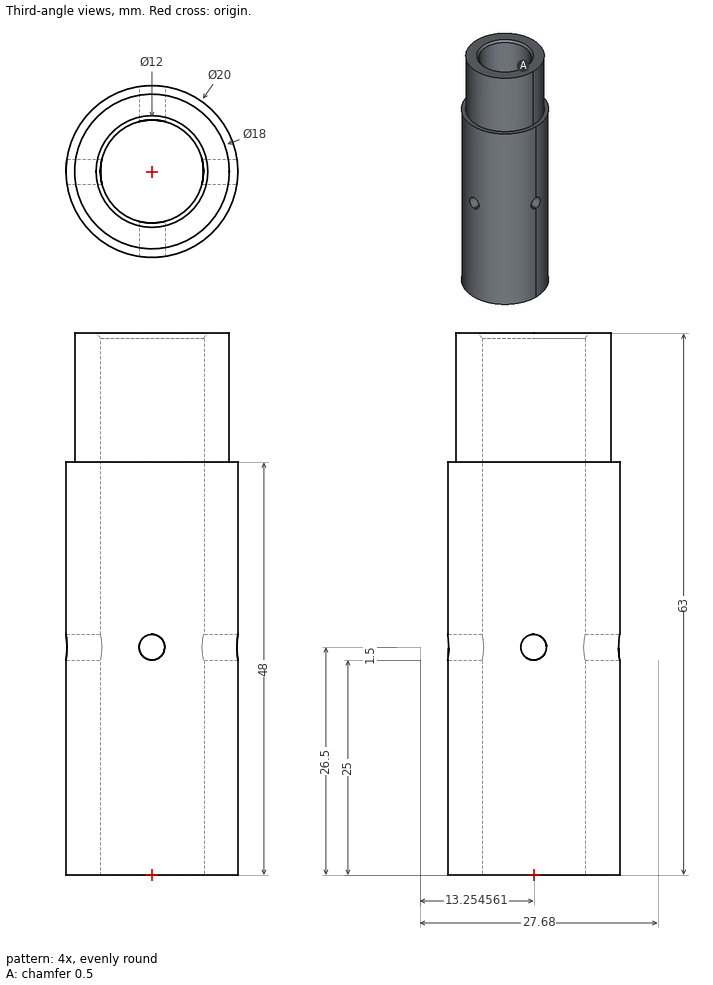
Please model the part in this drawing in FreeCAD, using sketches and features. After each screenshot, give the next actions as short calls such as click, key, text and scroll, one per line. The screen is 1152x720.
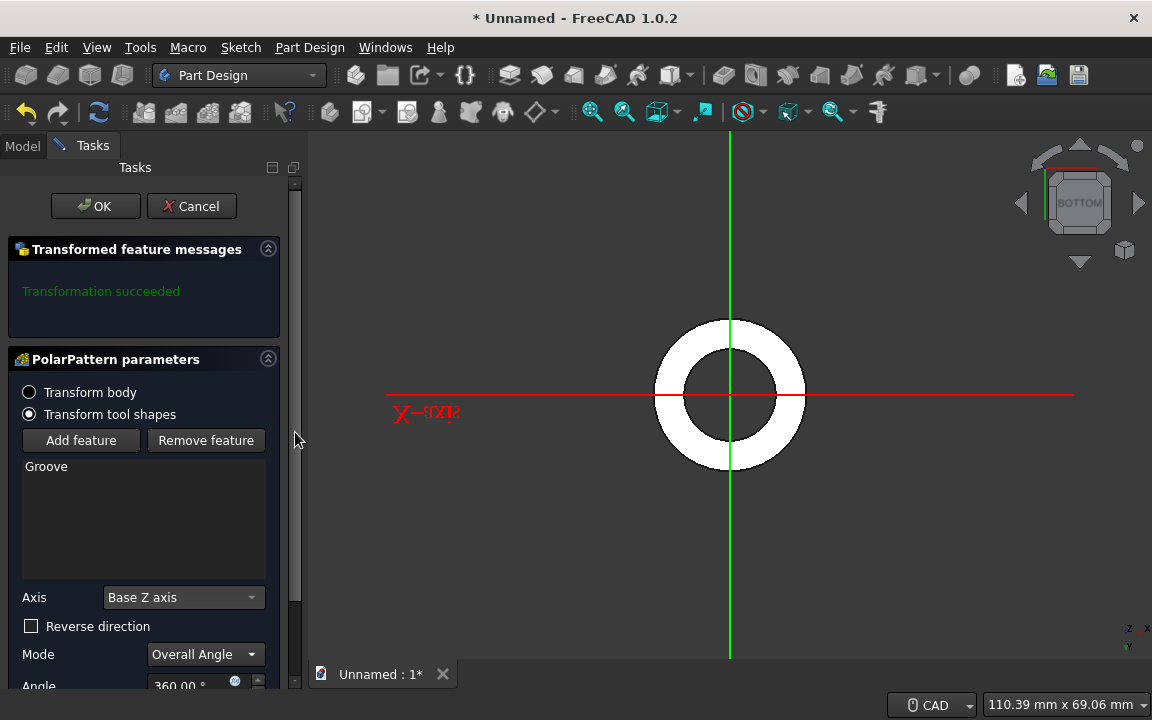
click(96, 206)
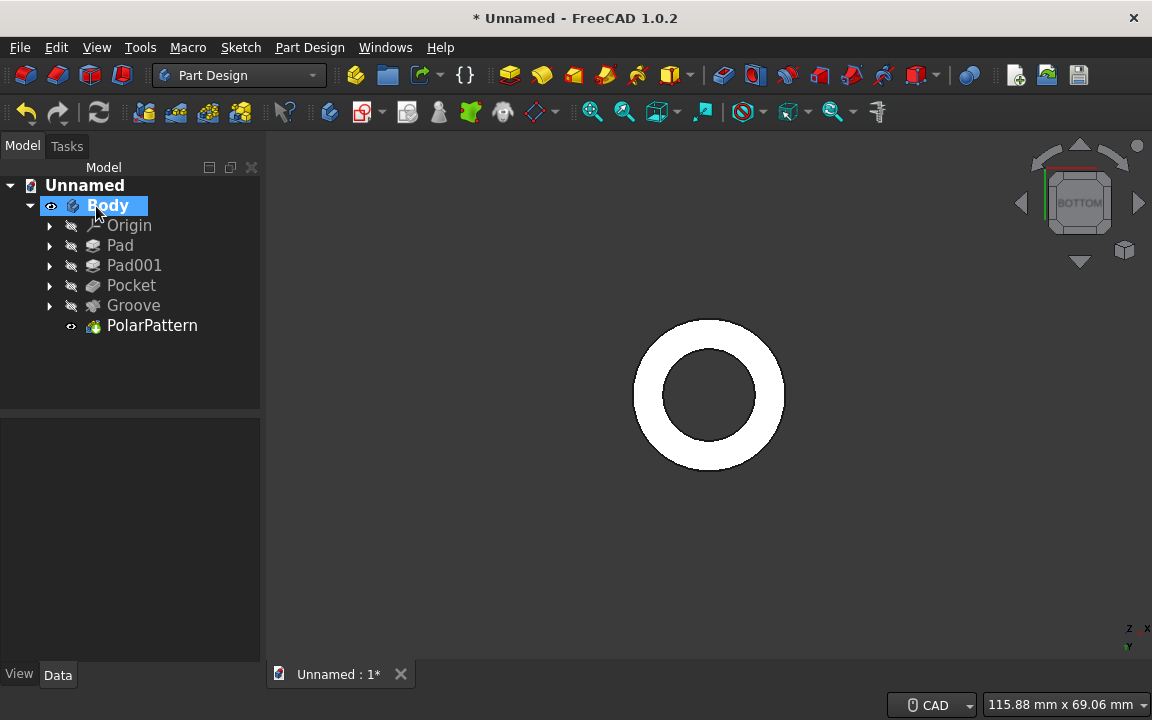
click(594, 112)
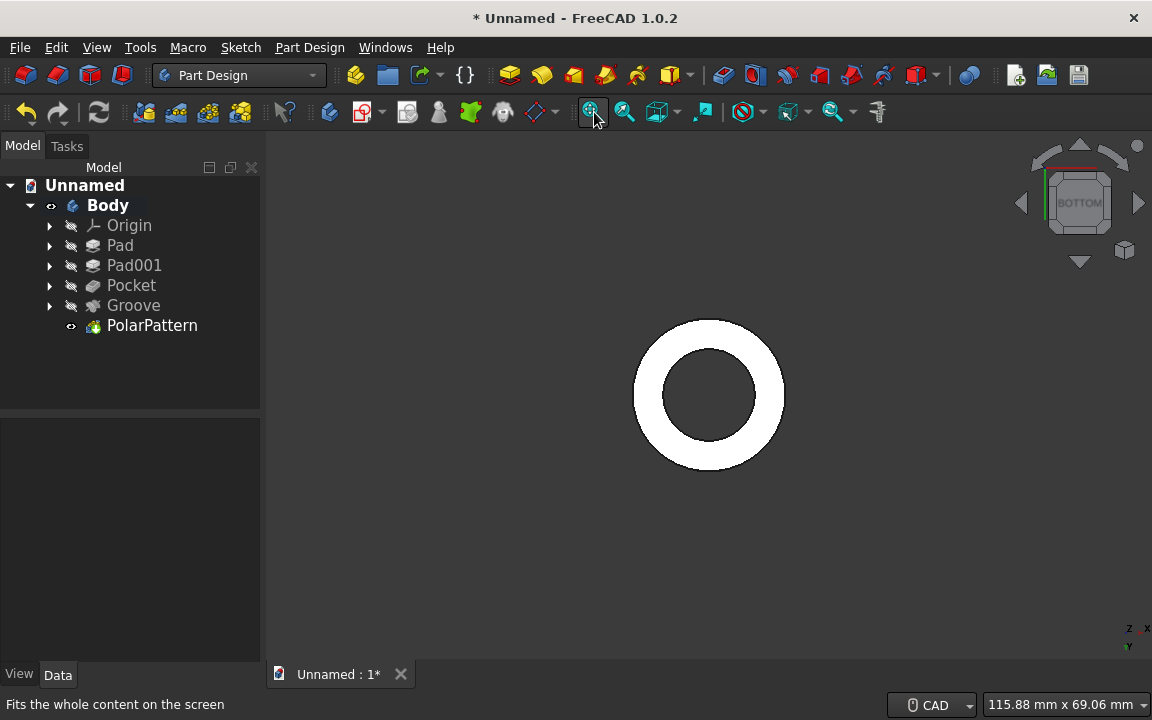
key(0)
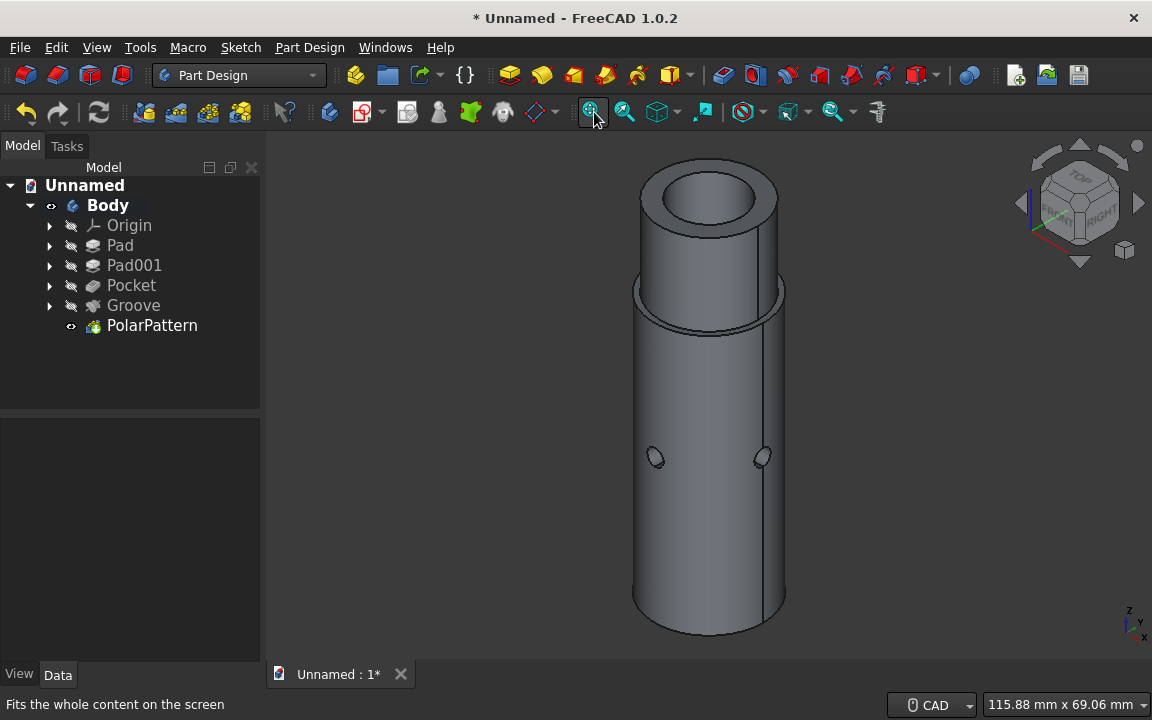
click(677, 179)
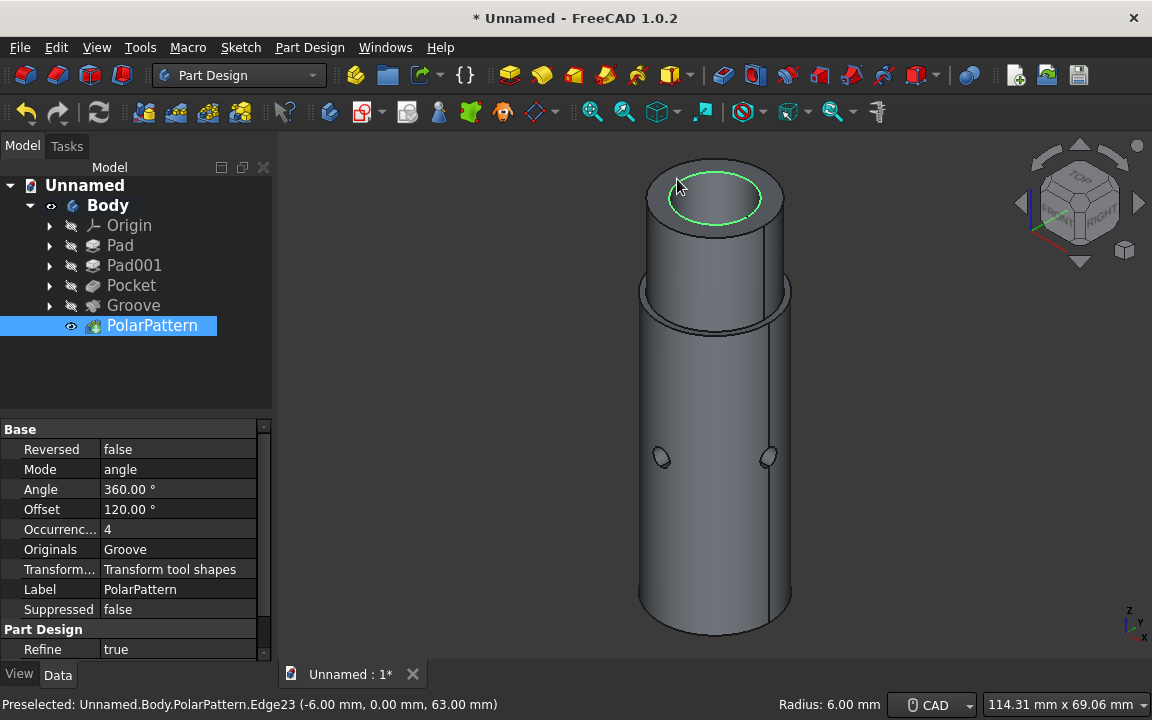
click(58, 76)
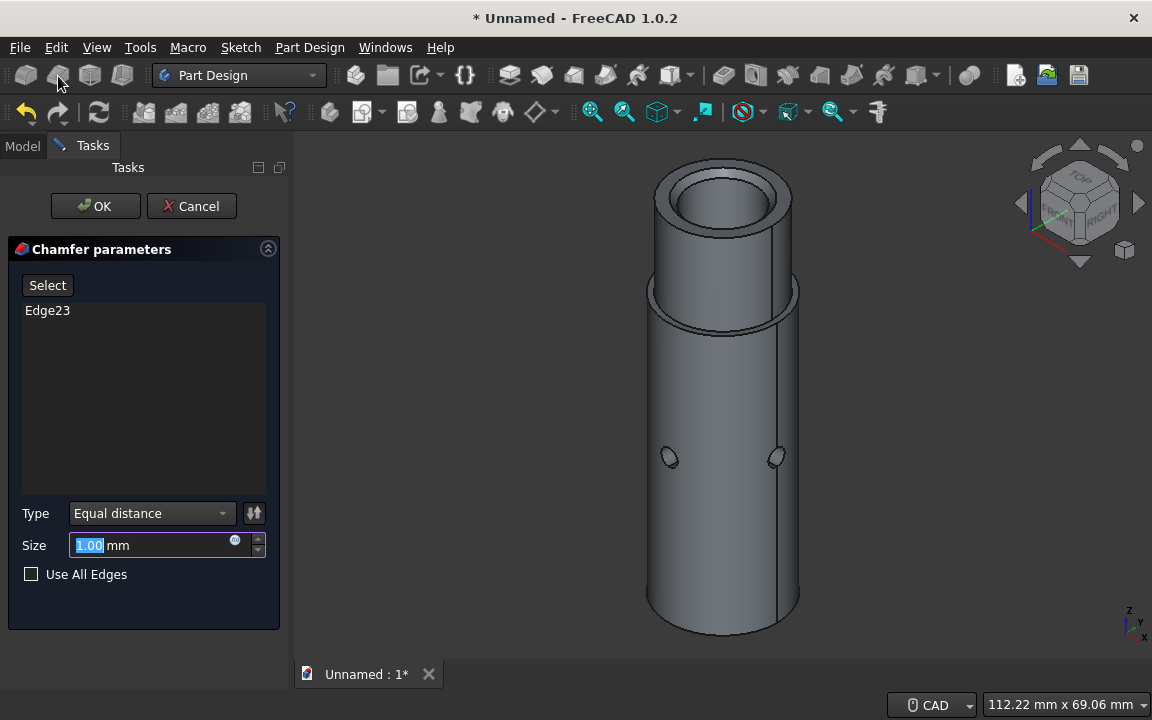
text(0.5)
key(Tab)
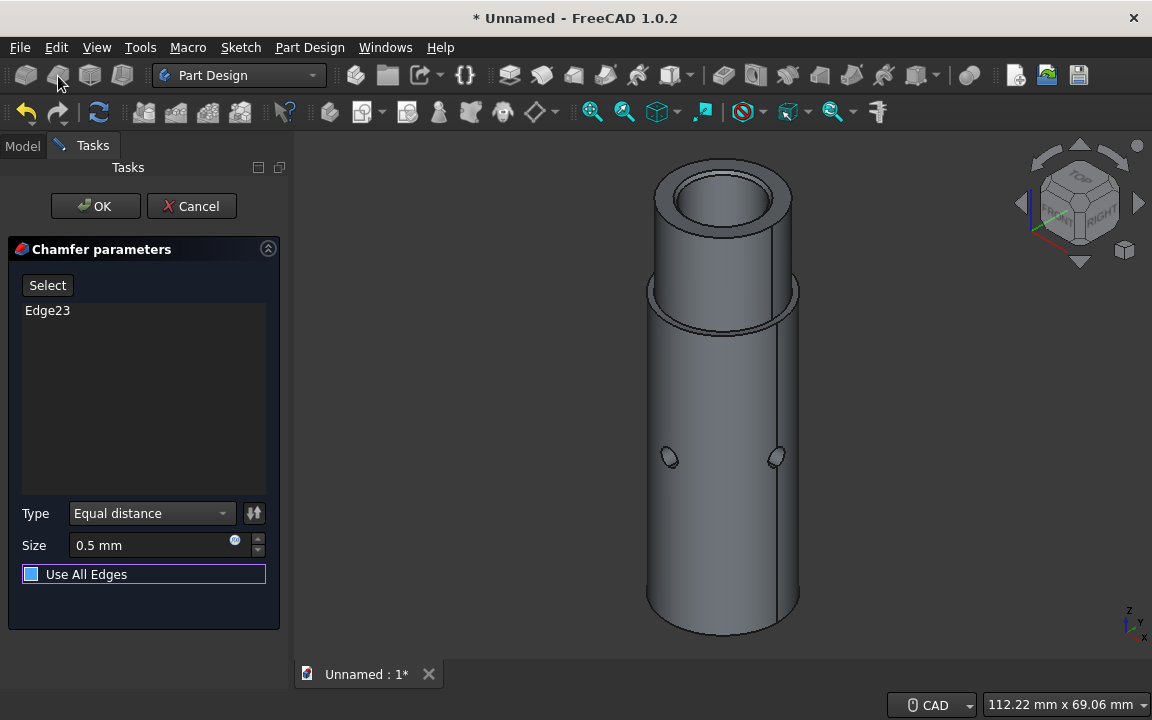
click(96, 206)